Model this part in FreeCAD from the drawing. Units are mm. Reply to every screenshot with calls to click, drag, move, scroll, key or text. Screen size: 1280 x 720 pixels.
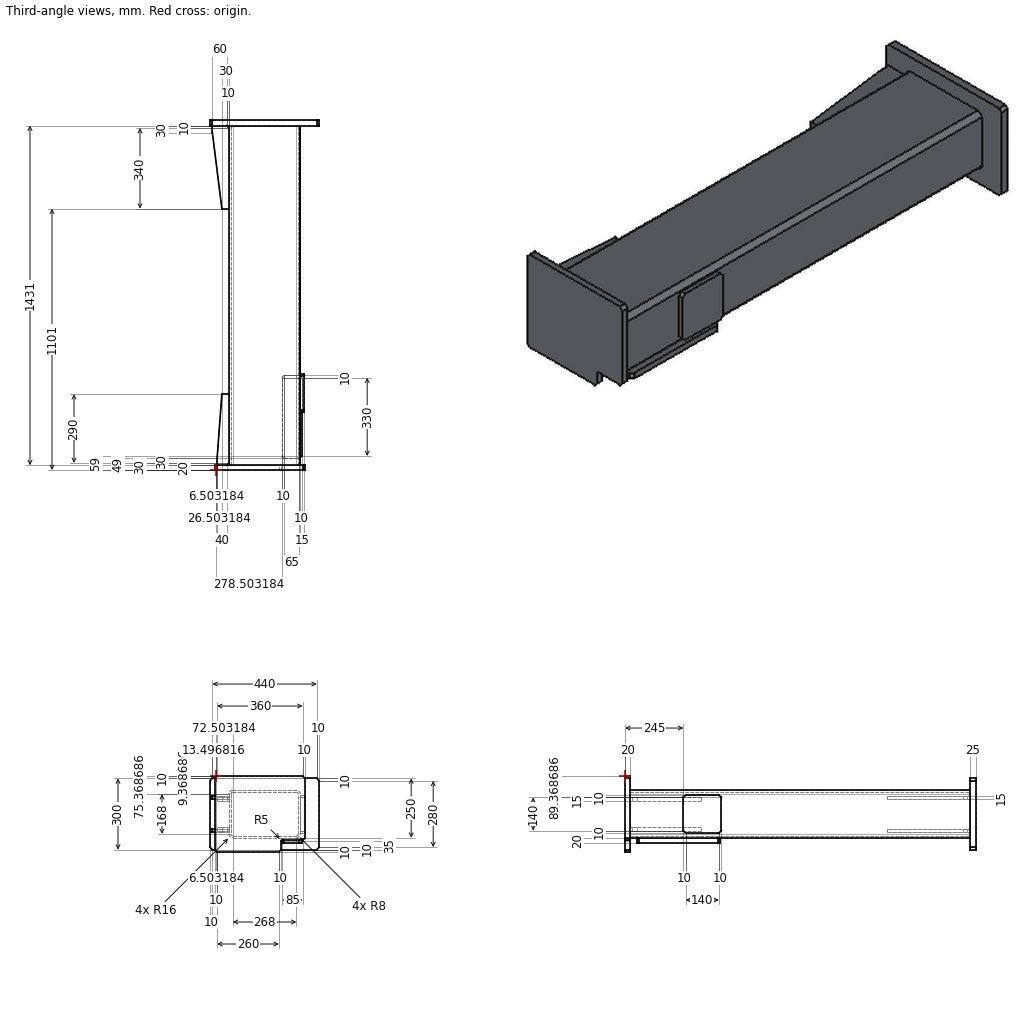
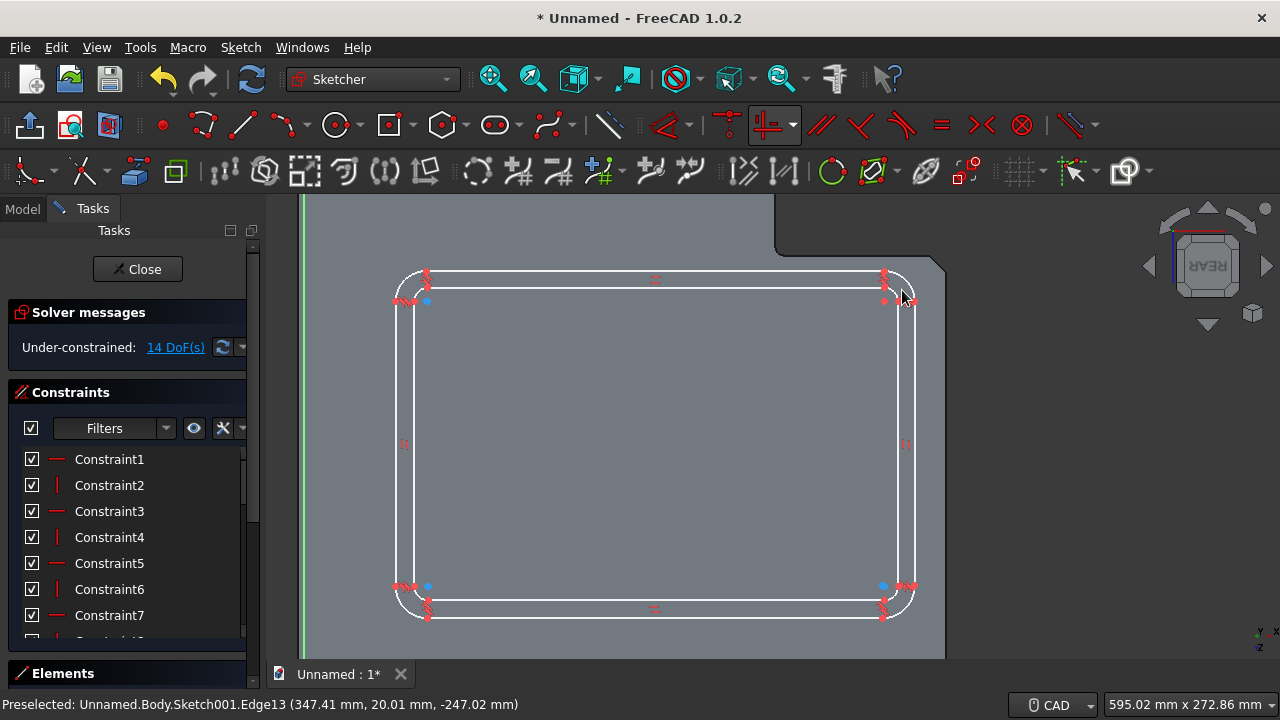
scroll(899, 508, up, 2)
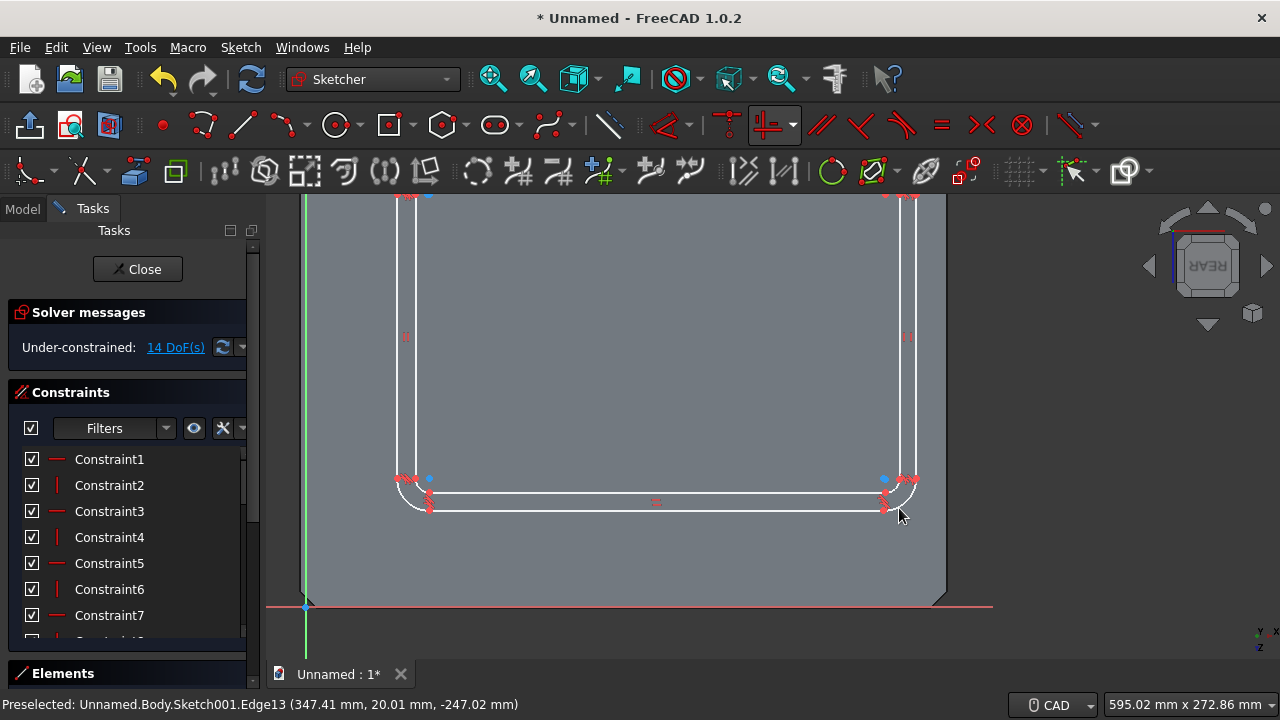
click(898, 507)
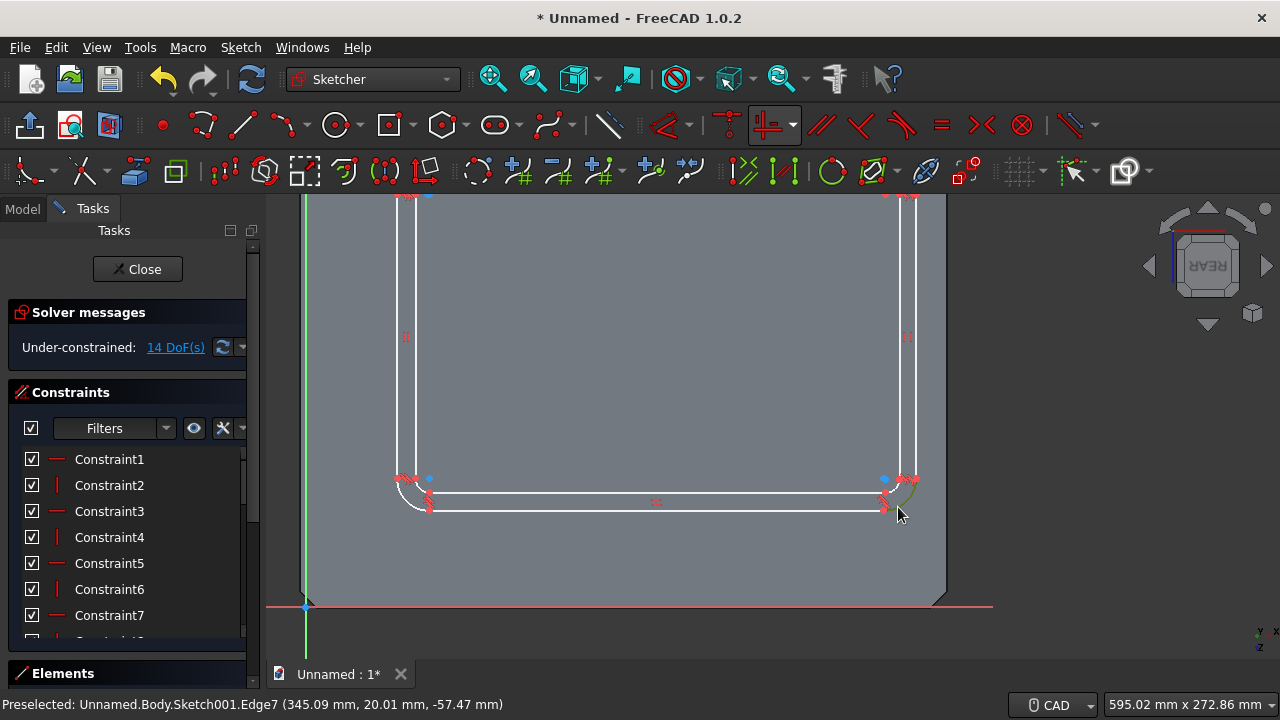
scroll(895, 489, up, 2)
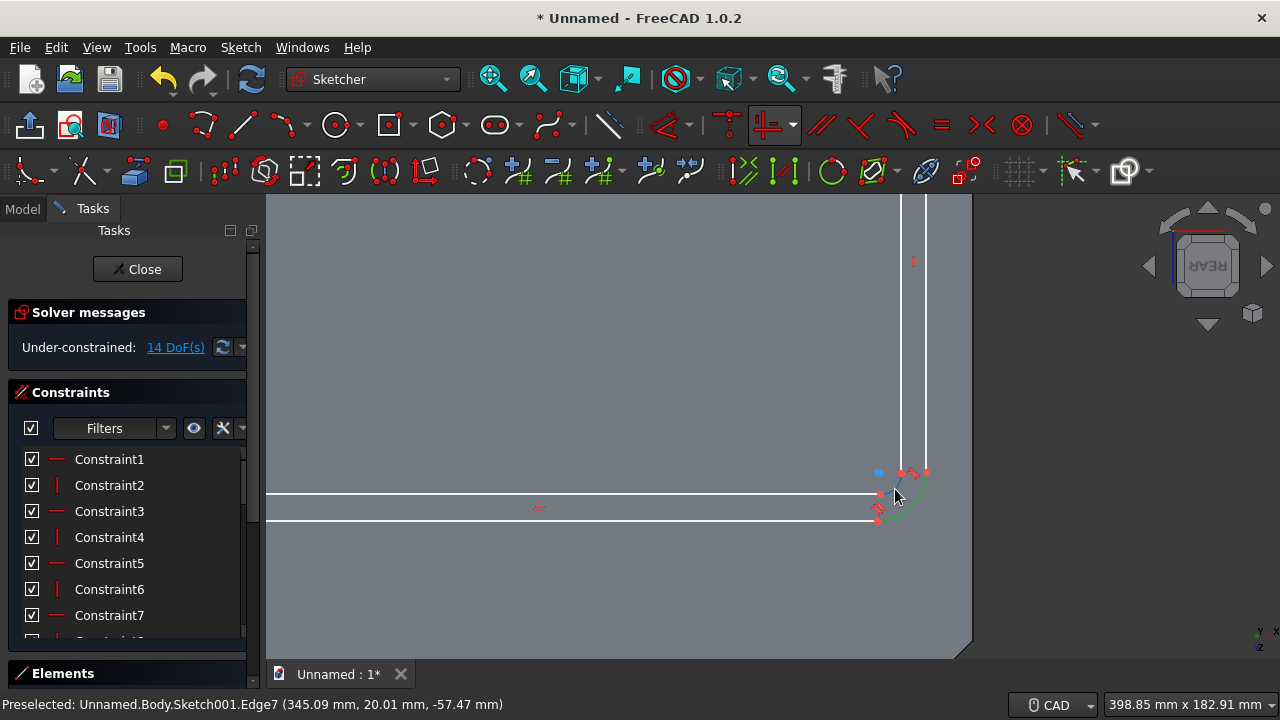
click(895, 488)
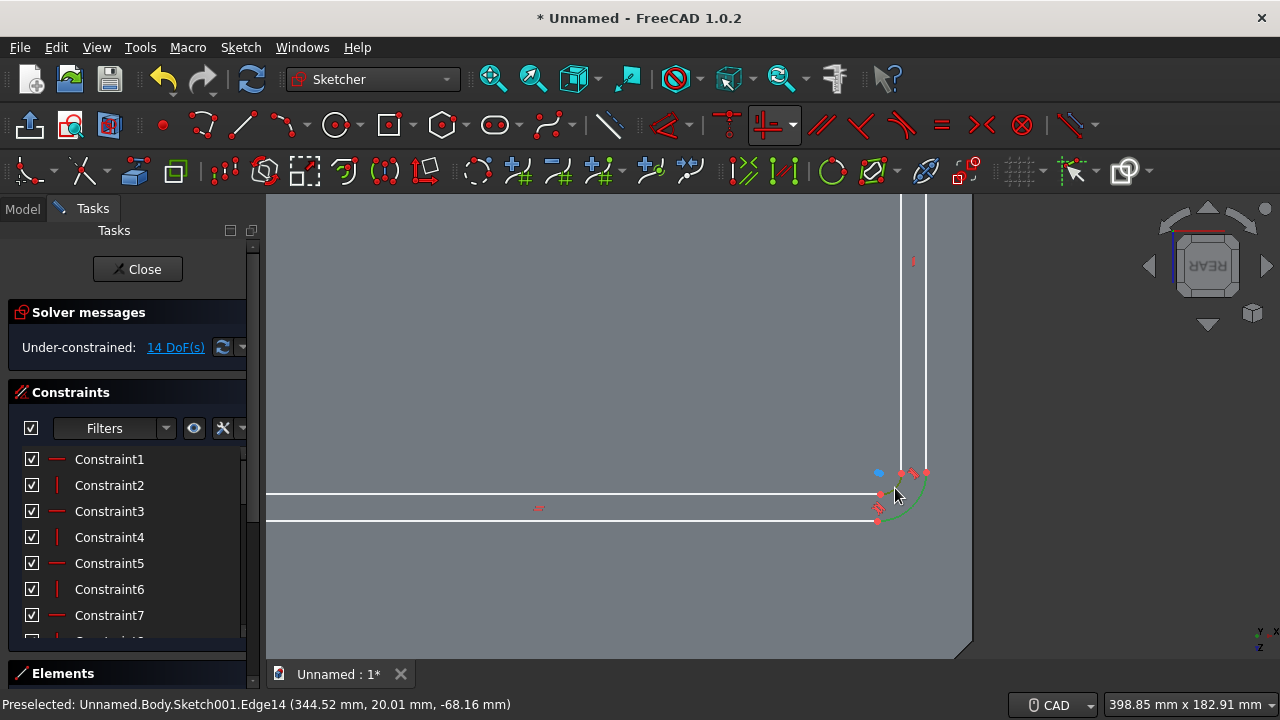
click(728, 126)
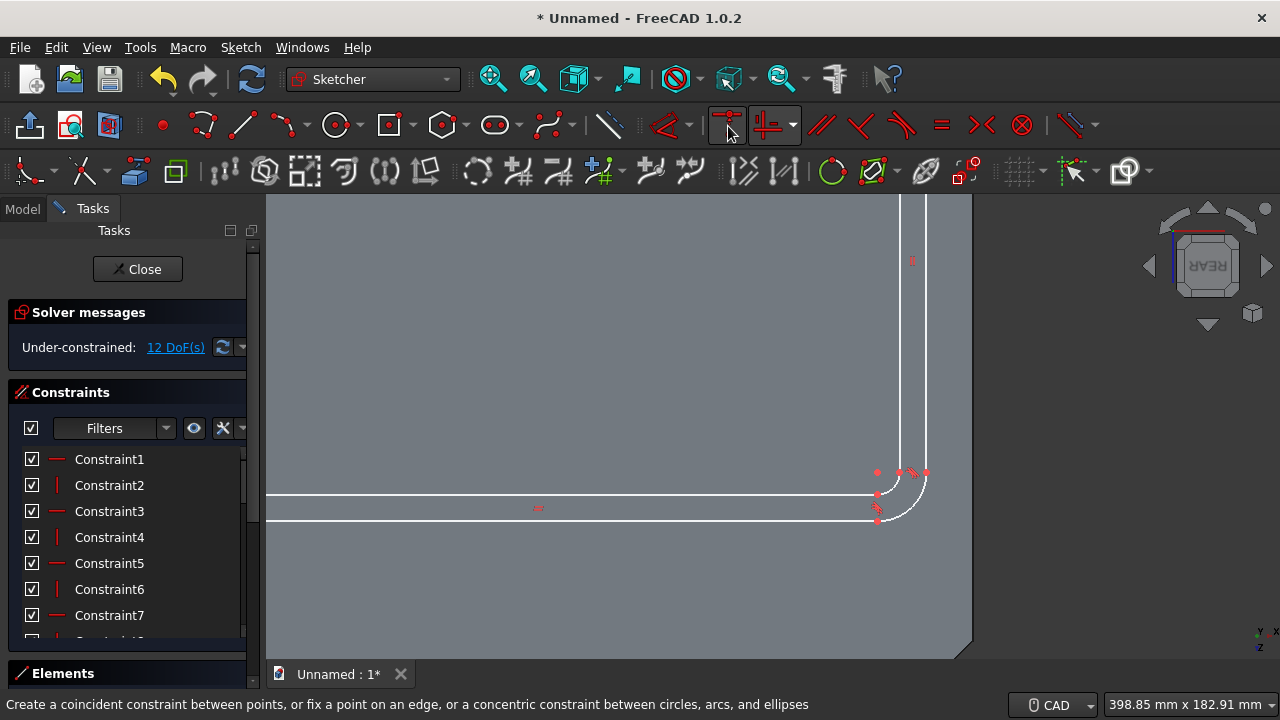
scroll(897, 501, down, 4)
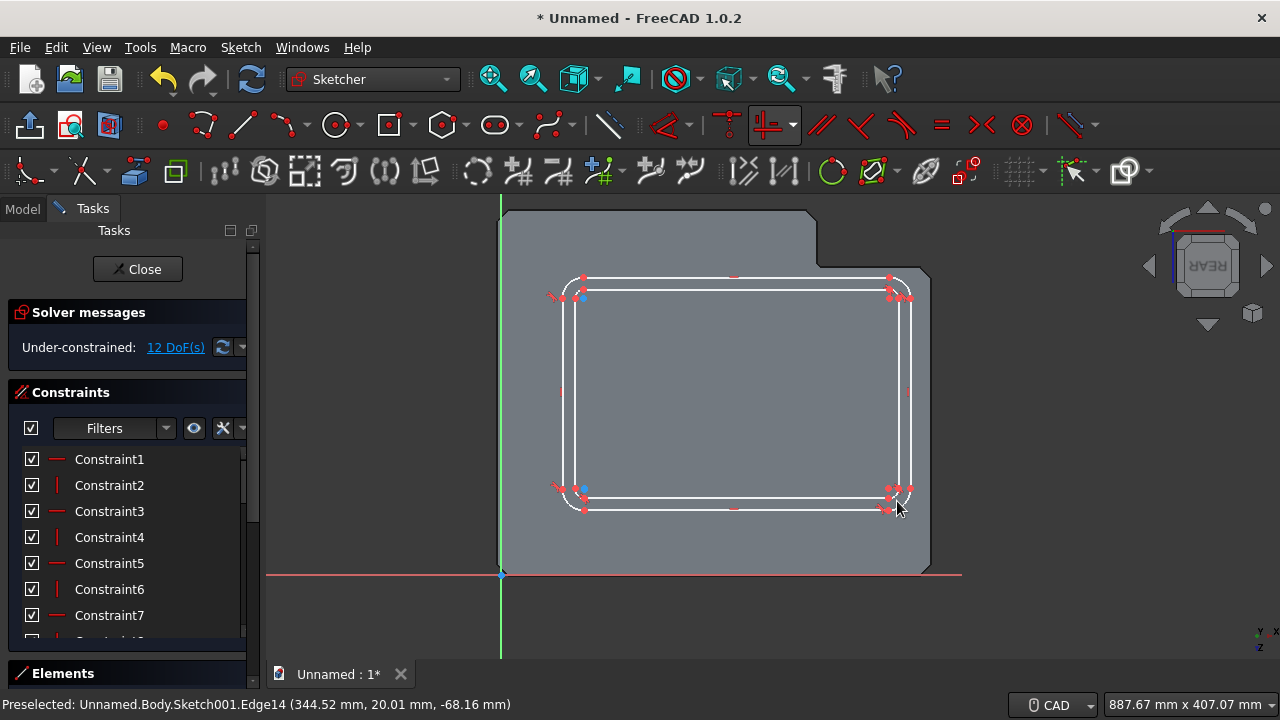
scroll(565, 499, up, 2)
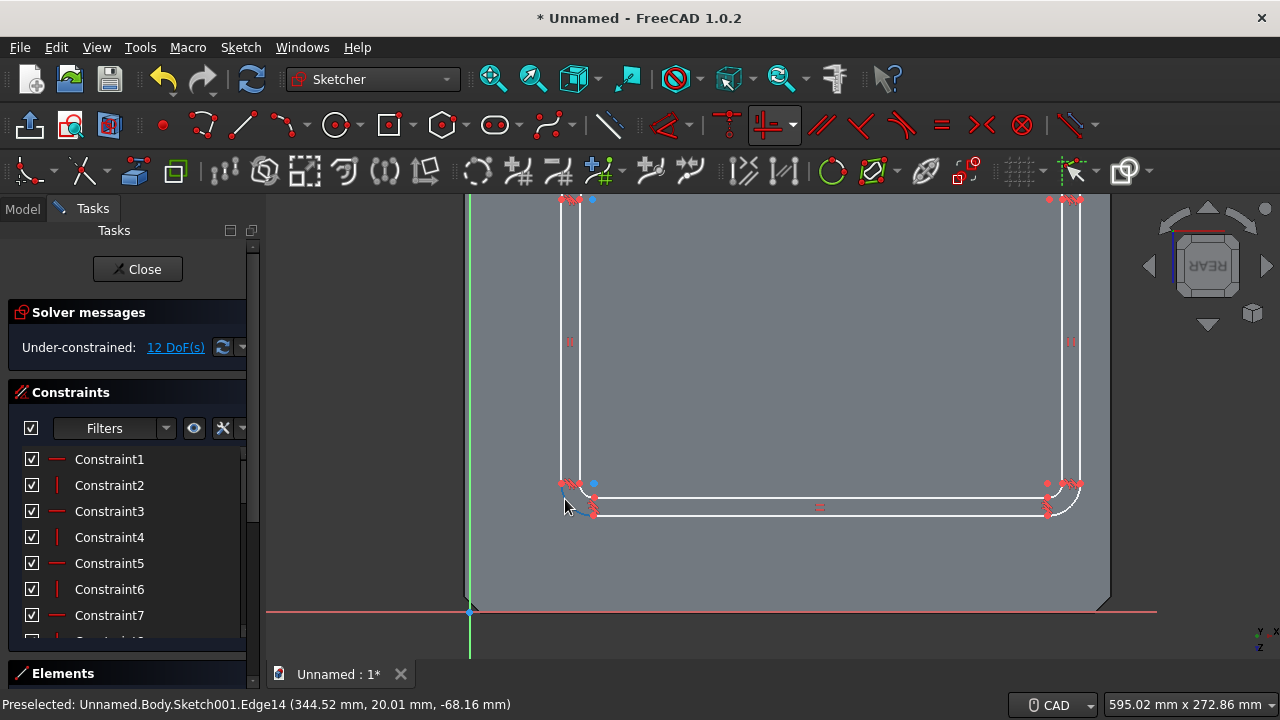
click(565, 498)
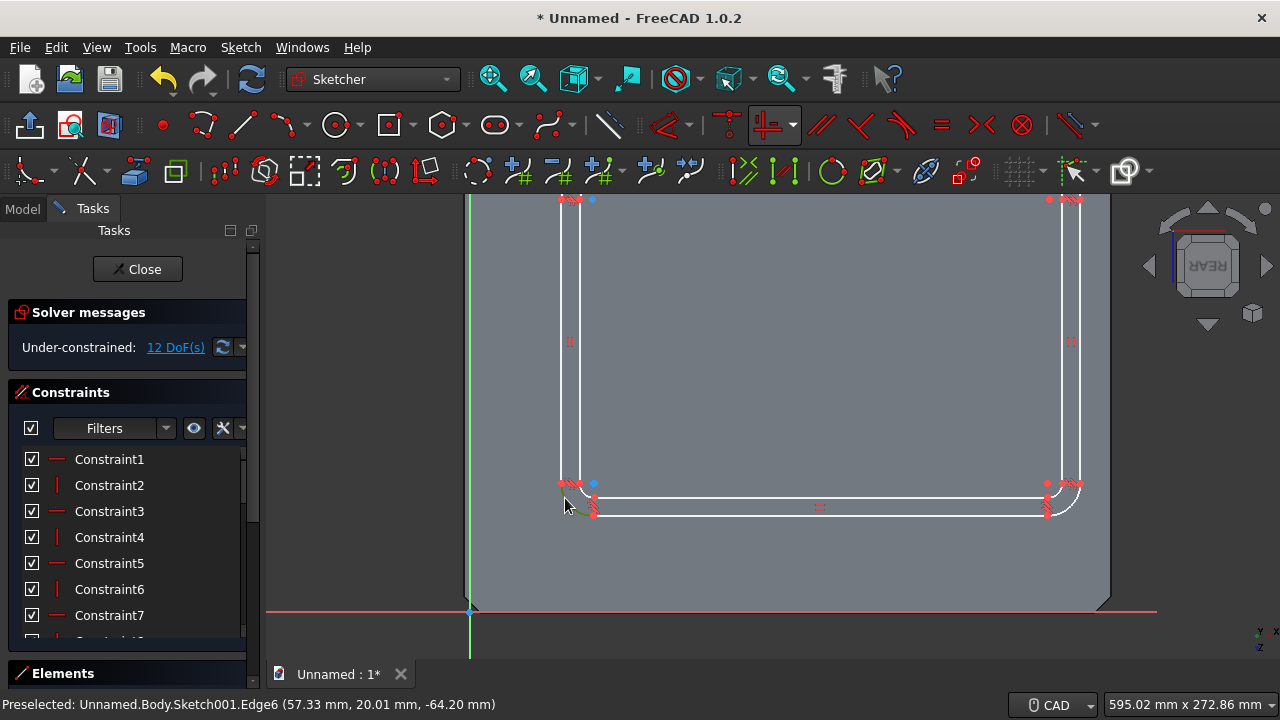
scroll(584, 494, up, 2)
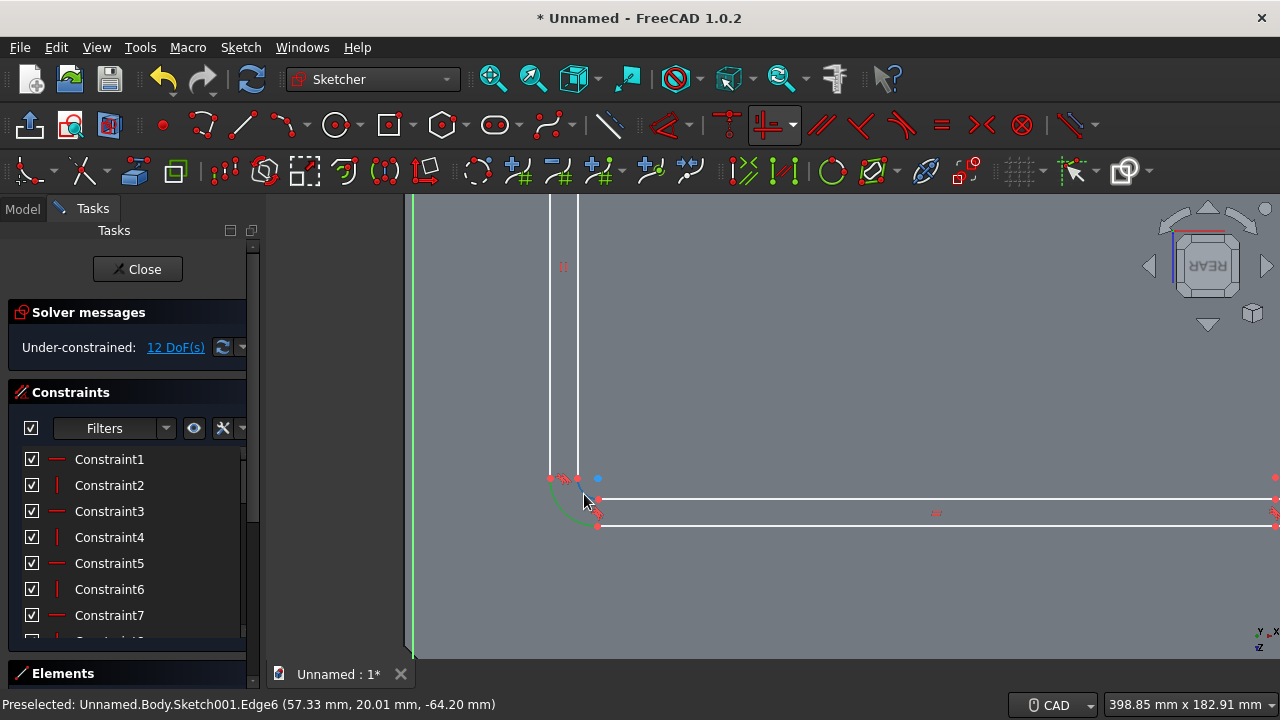
click(584, 493)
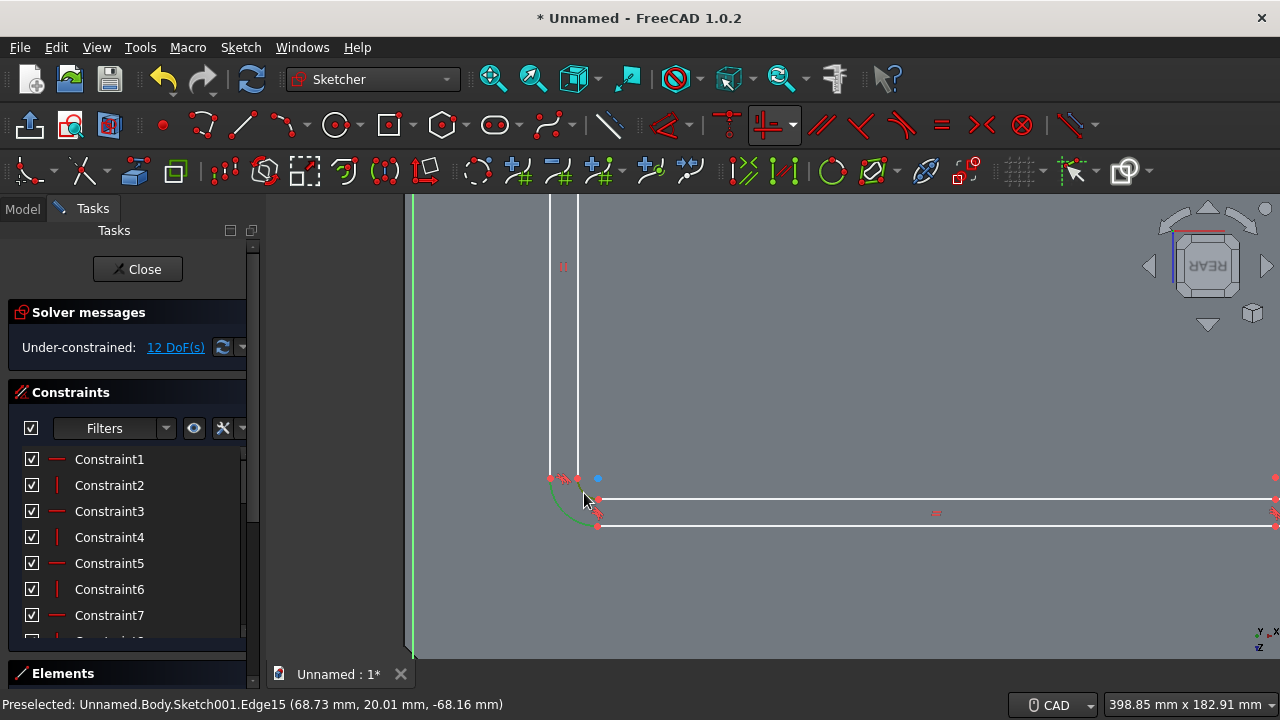
click(728, 126)